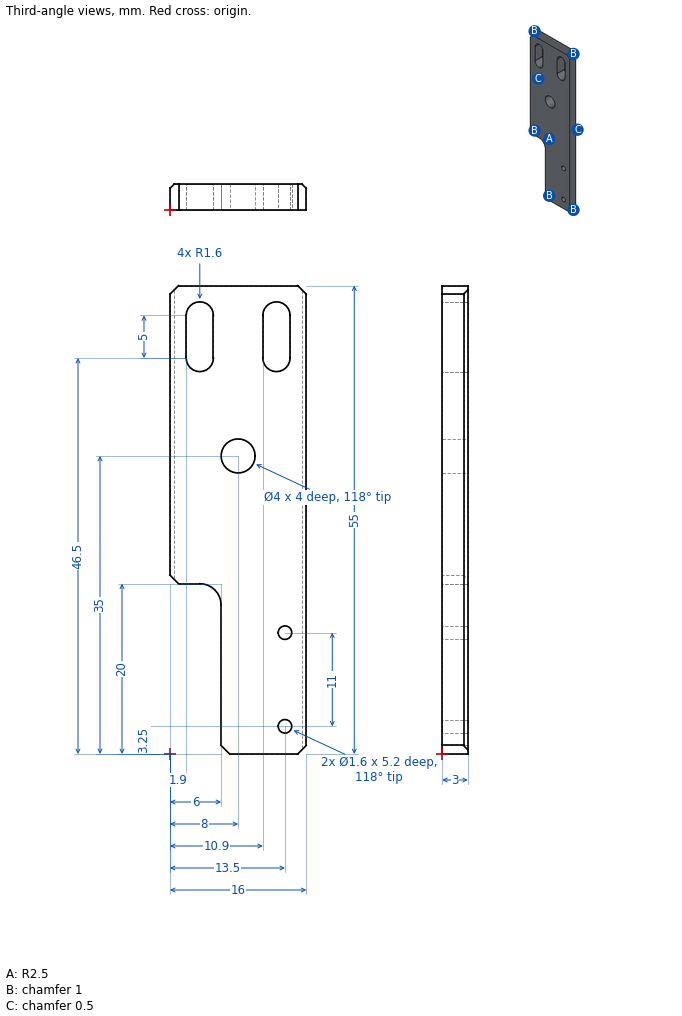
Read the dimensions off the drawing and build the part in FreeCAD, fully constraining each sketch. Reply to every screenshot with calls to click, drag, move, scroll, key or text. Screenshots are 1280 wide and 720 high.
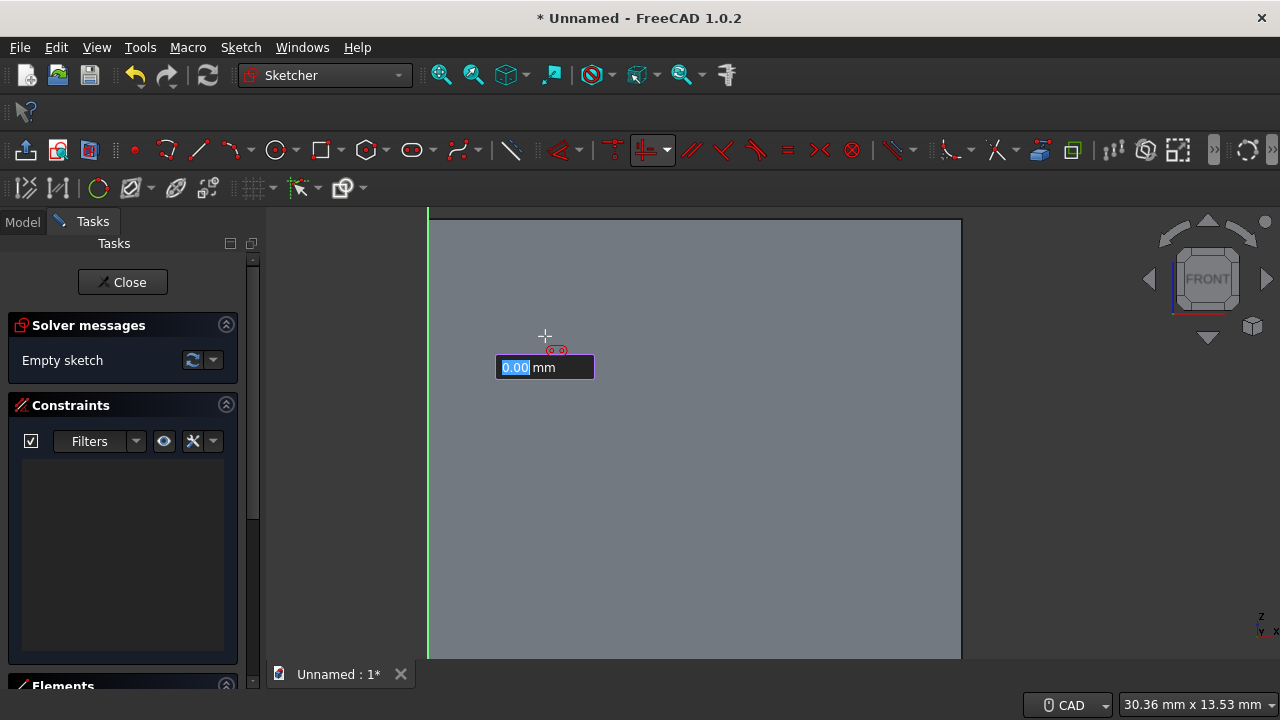
click(598, 419)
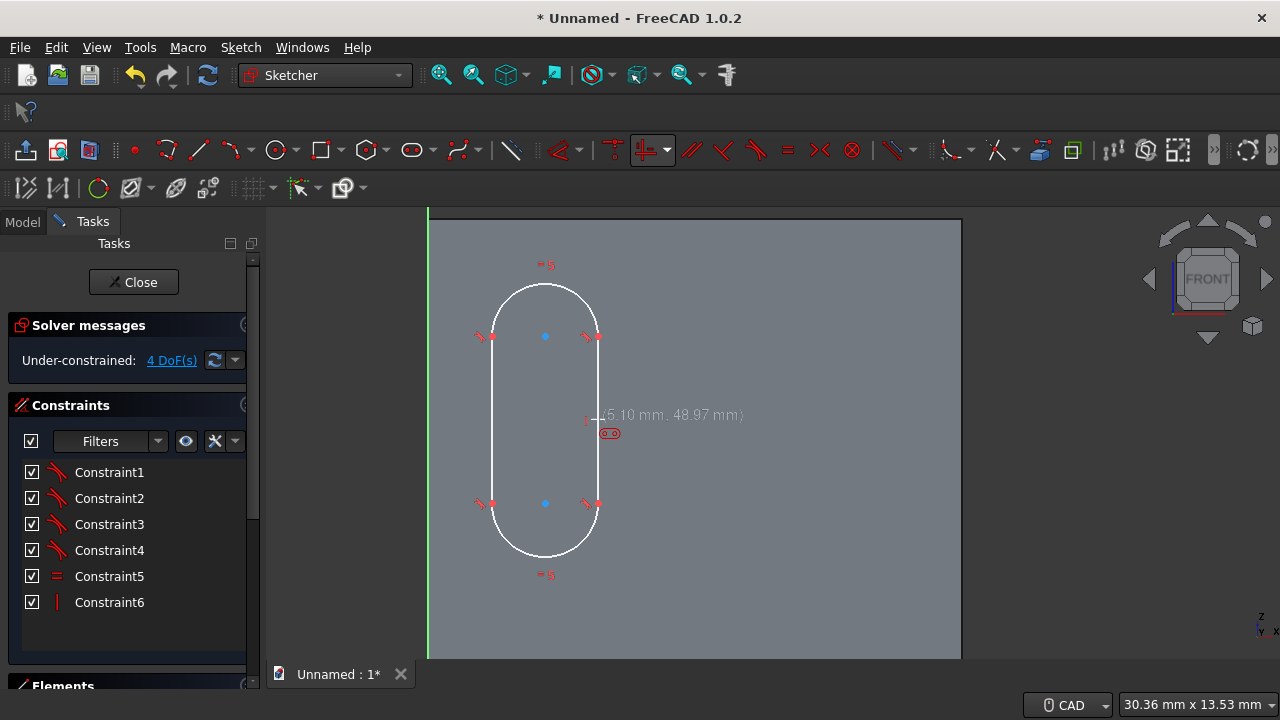
click(845, 503)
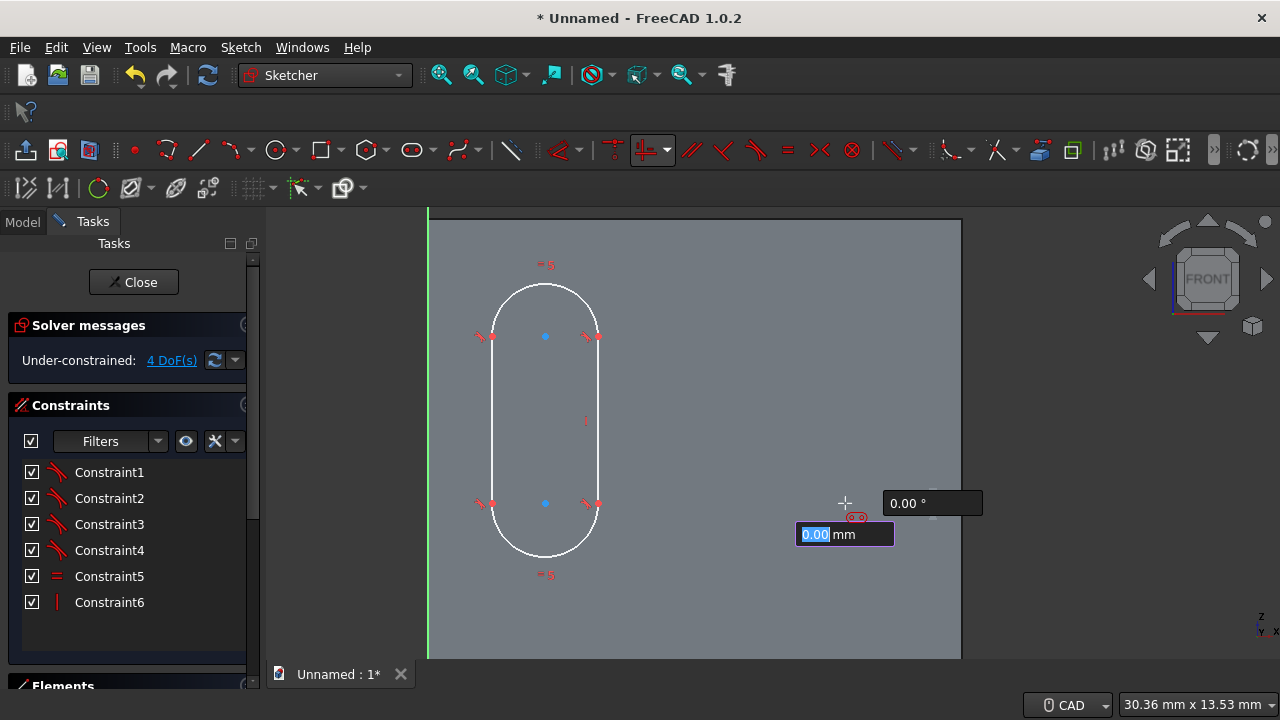
click(845, 336)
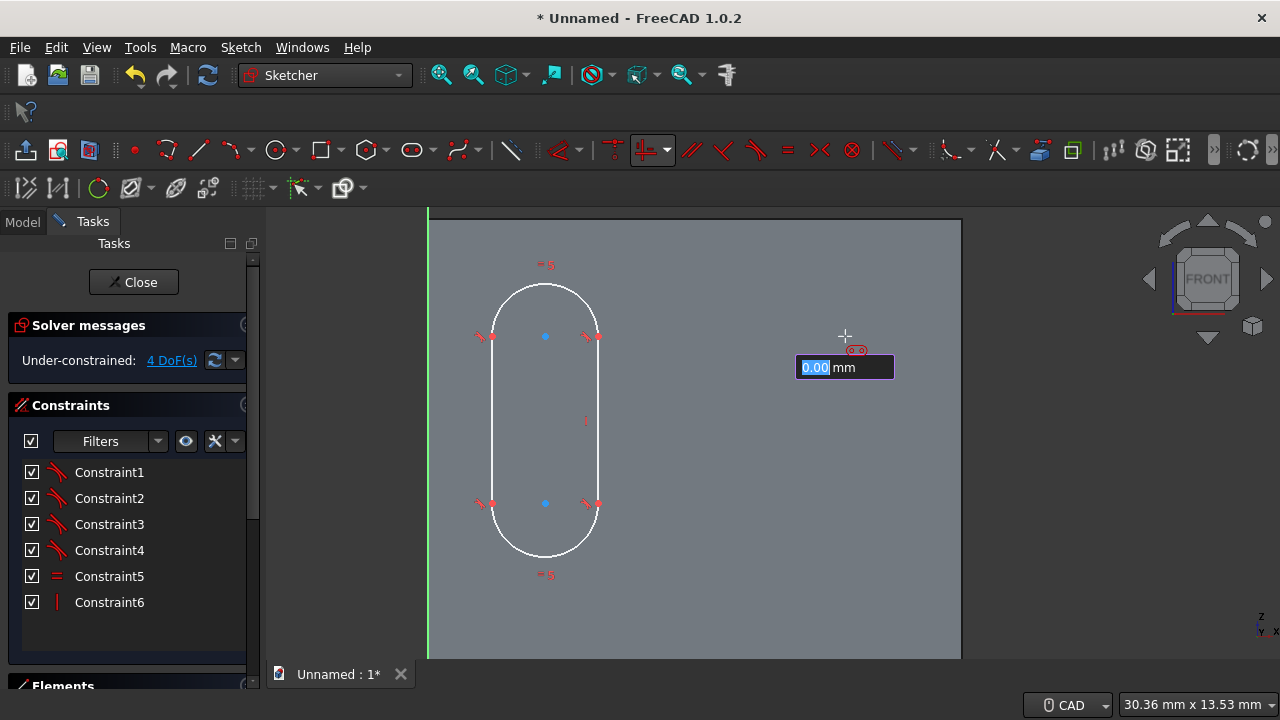
click(792, 419)
key(Escape)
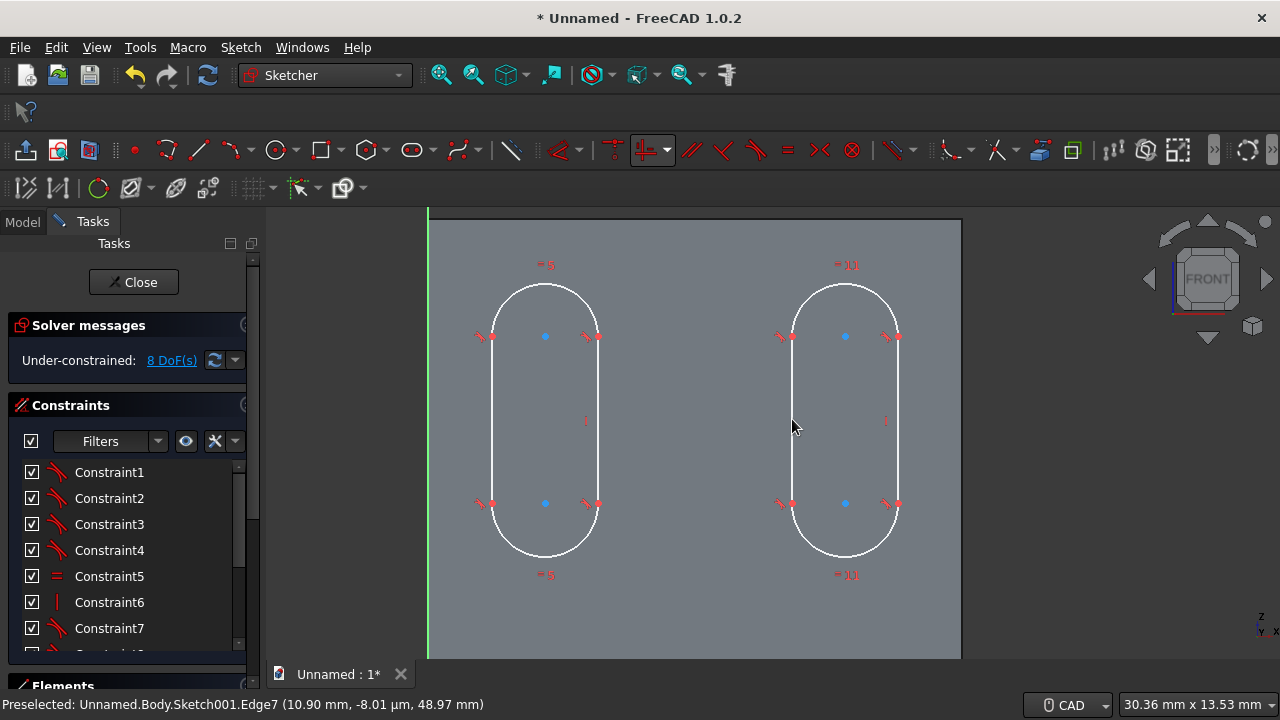
click(514, 547)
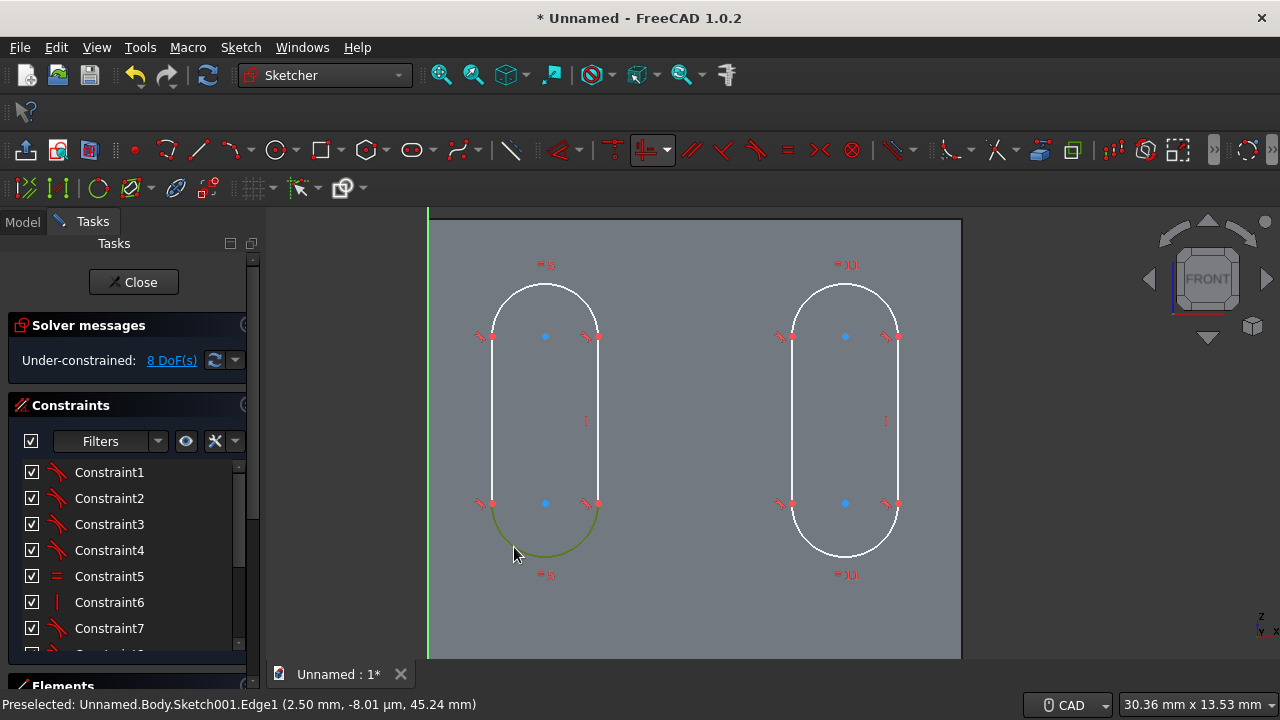
click(814, 547)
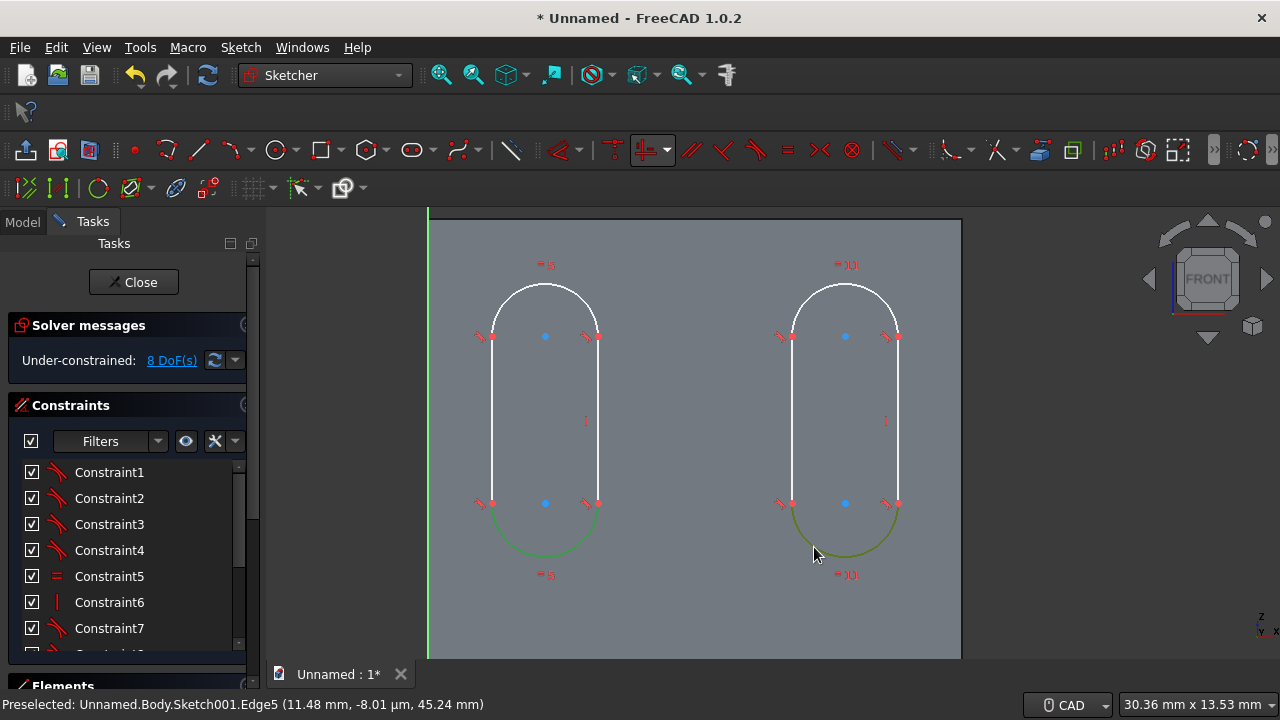
click(788, 150)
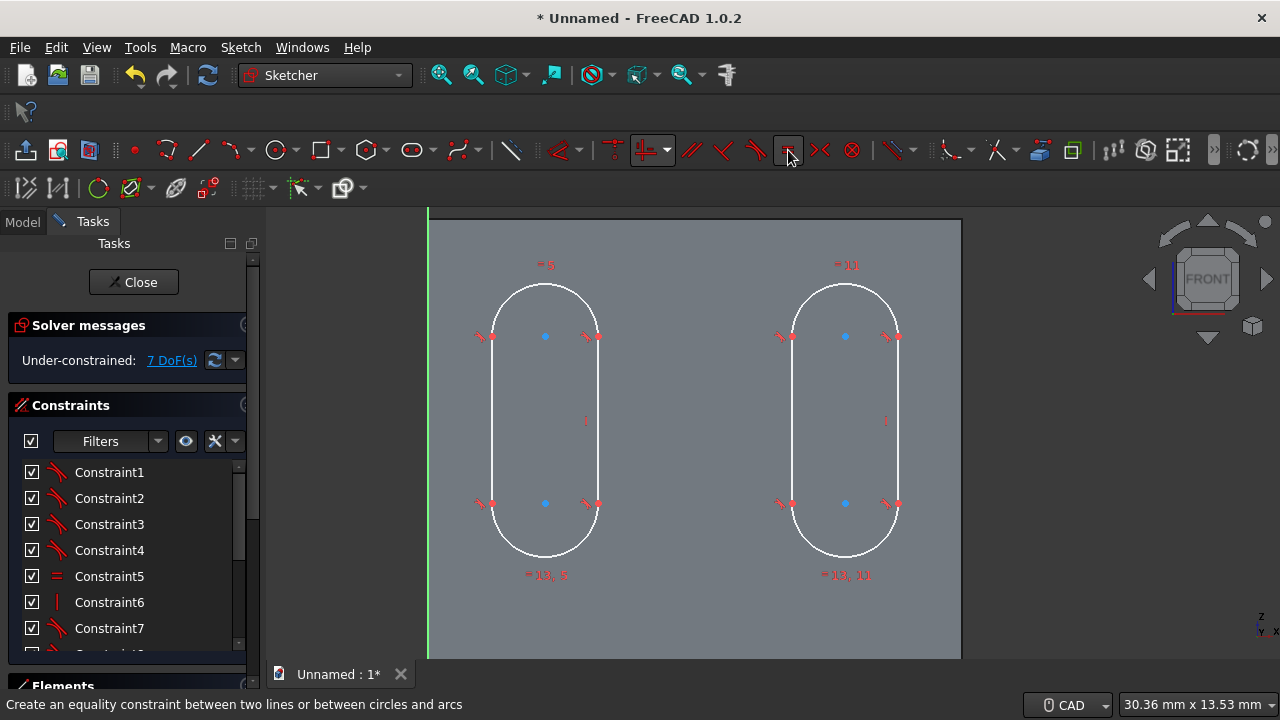
click(558, 150)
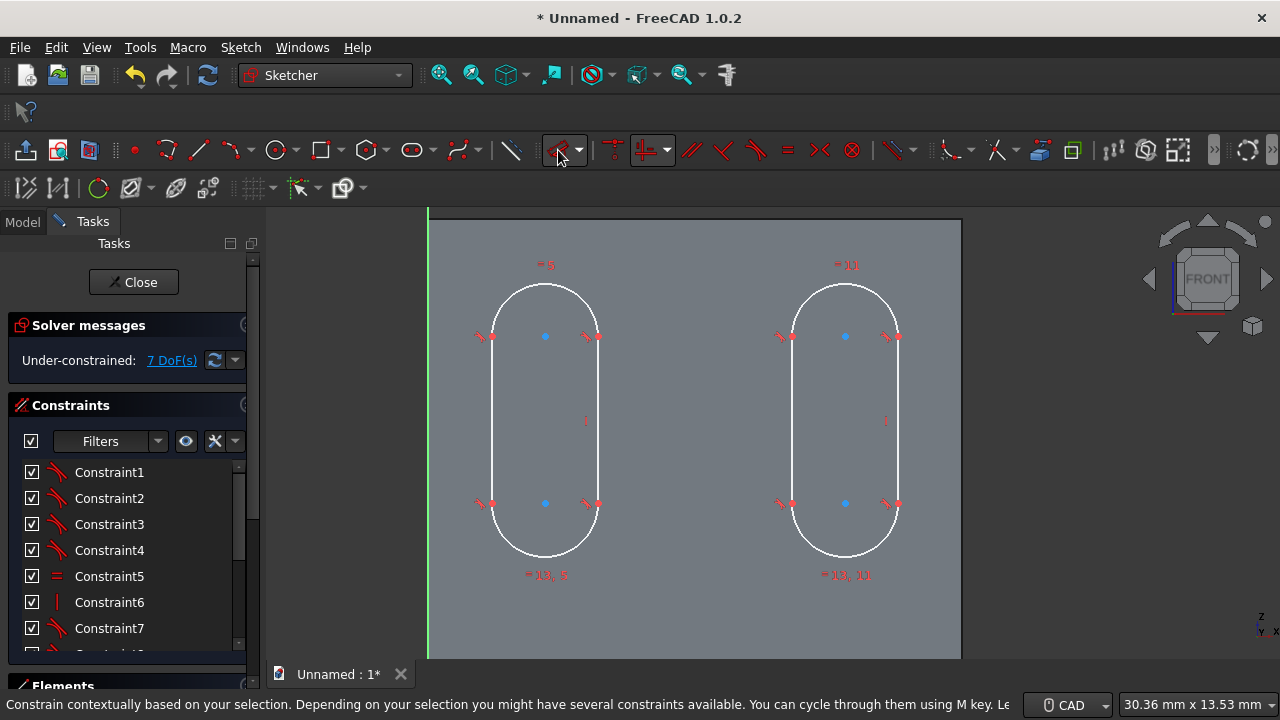
click(514, 547)
click(495, 573)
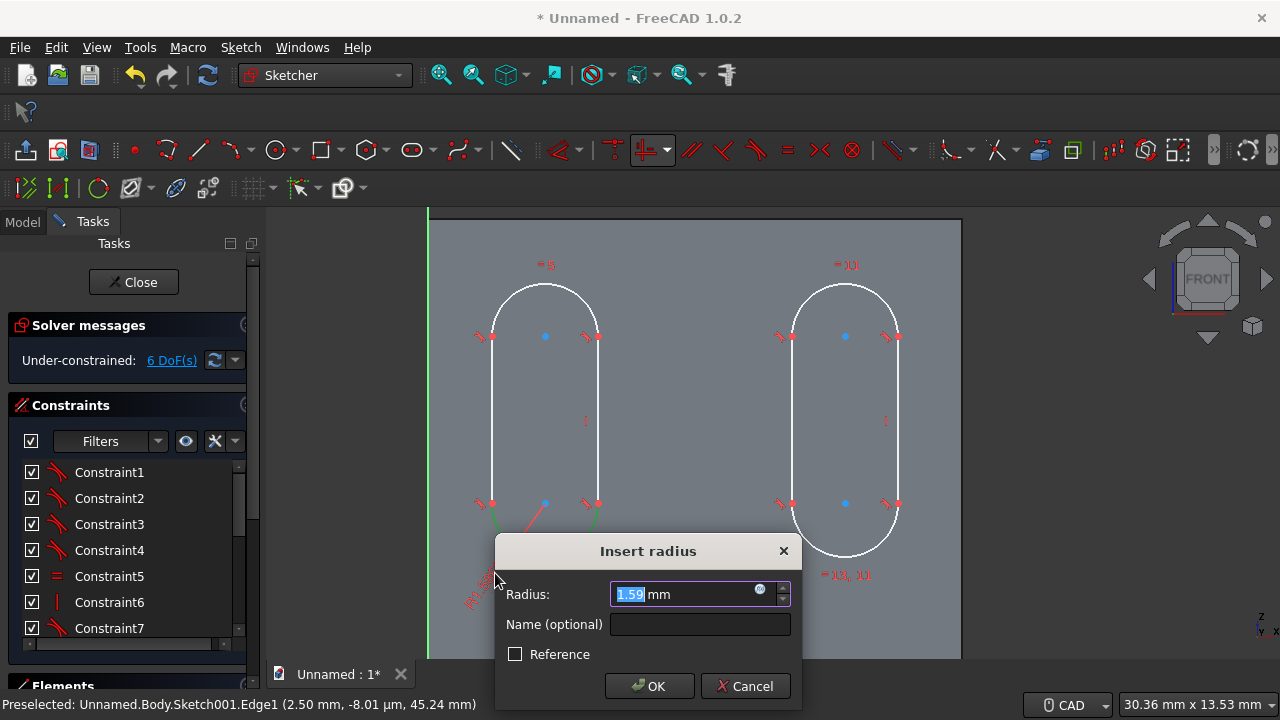
text(1.6)
key(Return)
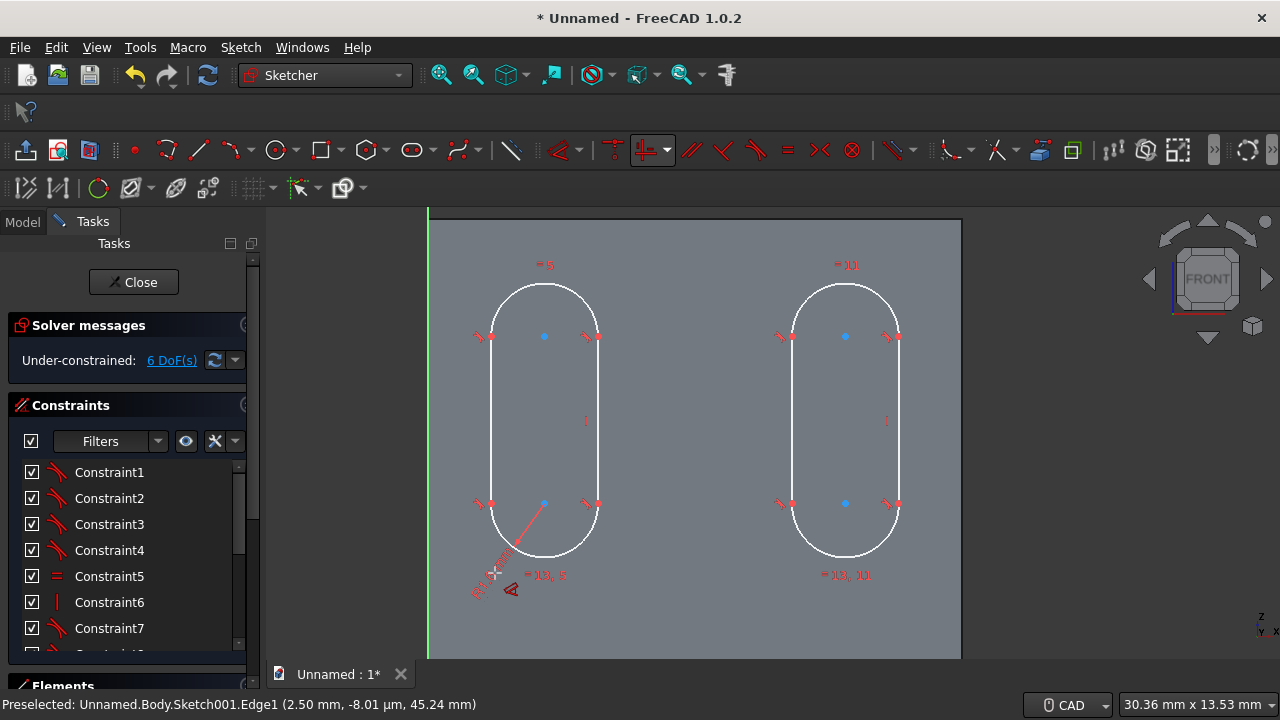
click(491, 454)
click(457, 421)